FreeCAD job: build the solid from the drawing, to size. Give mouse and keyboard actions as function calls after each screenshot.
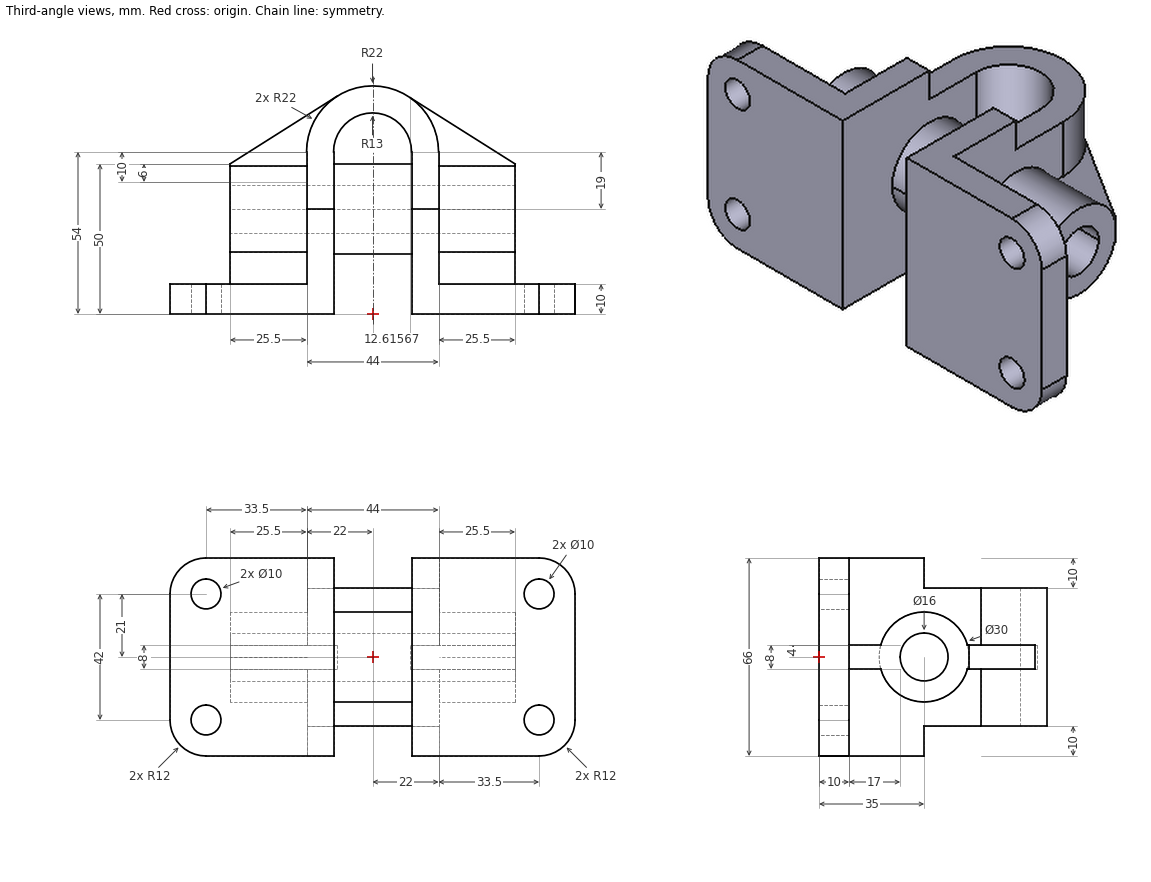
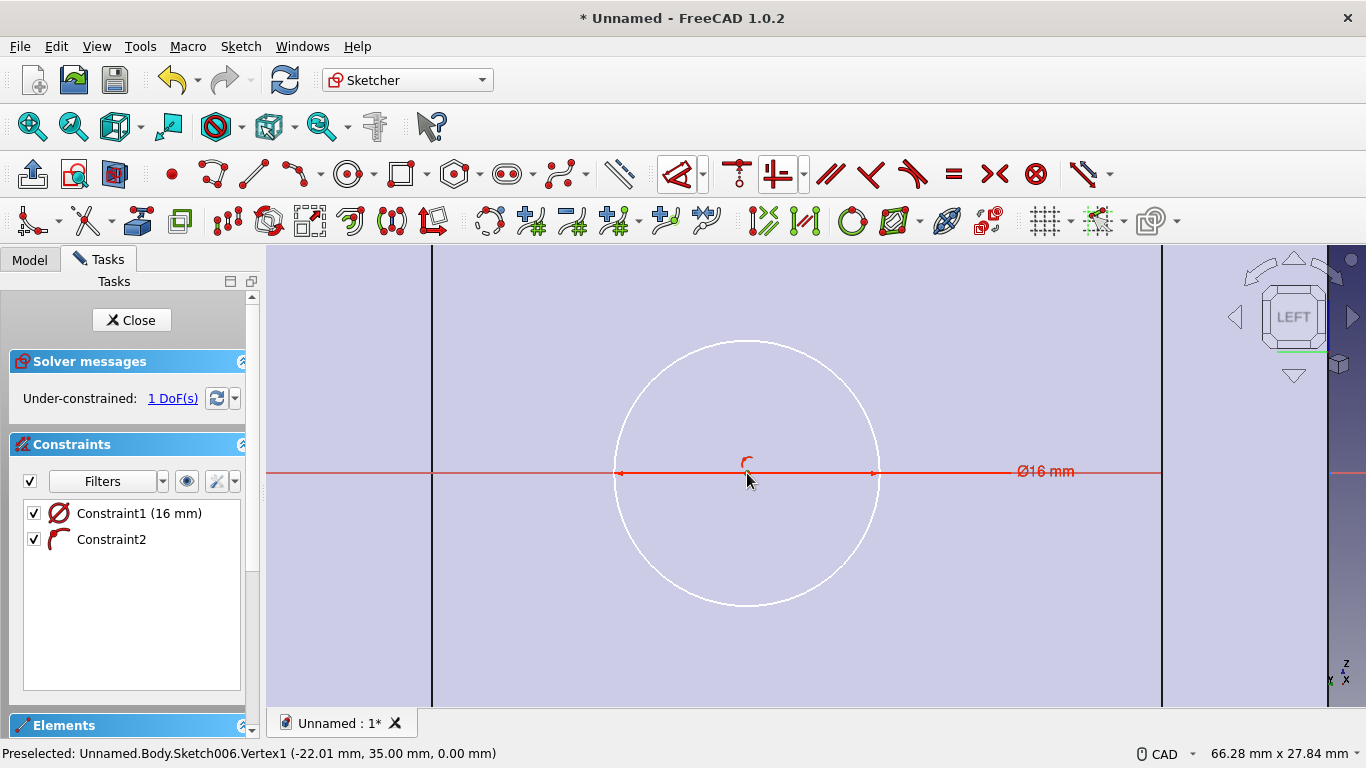
click(702, 174)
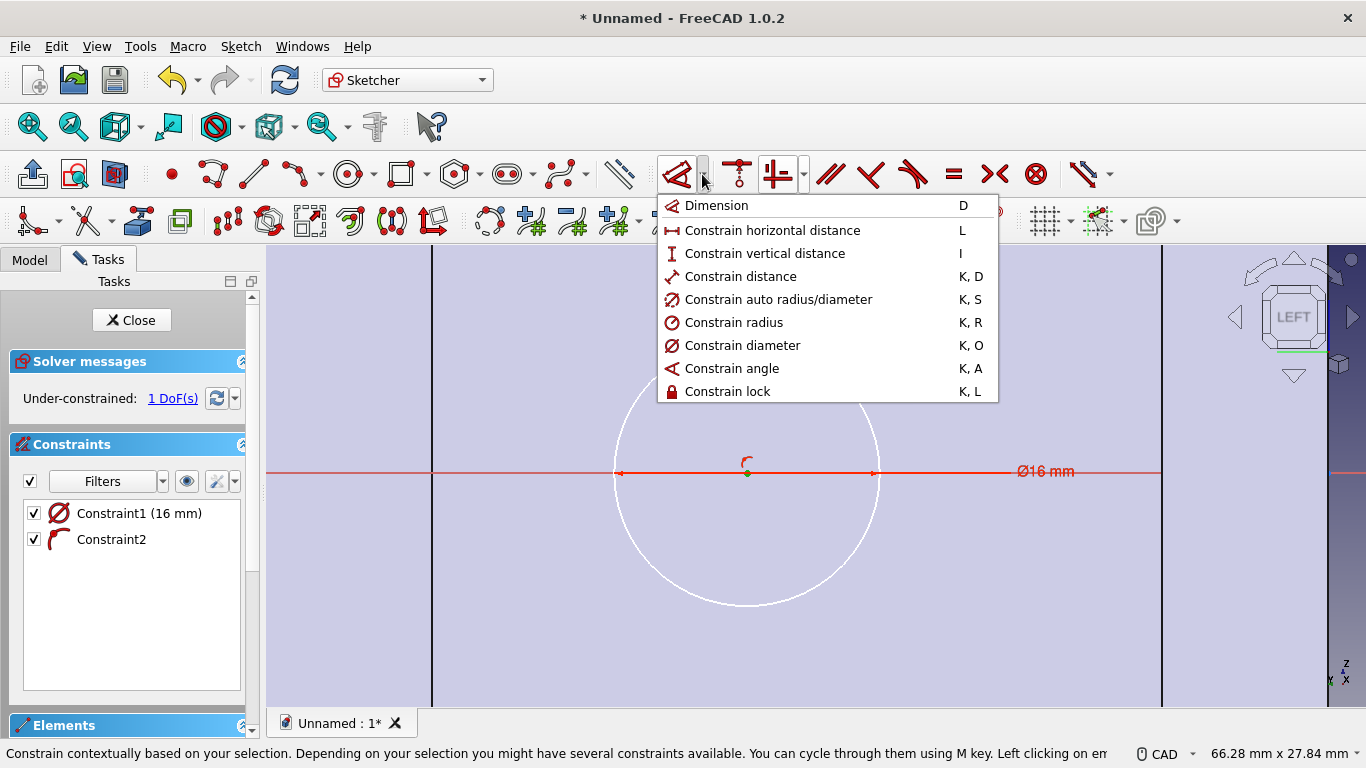
click(828, 230)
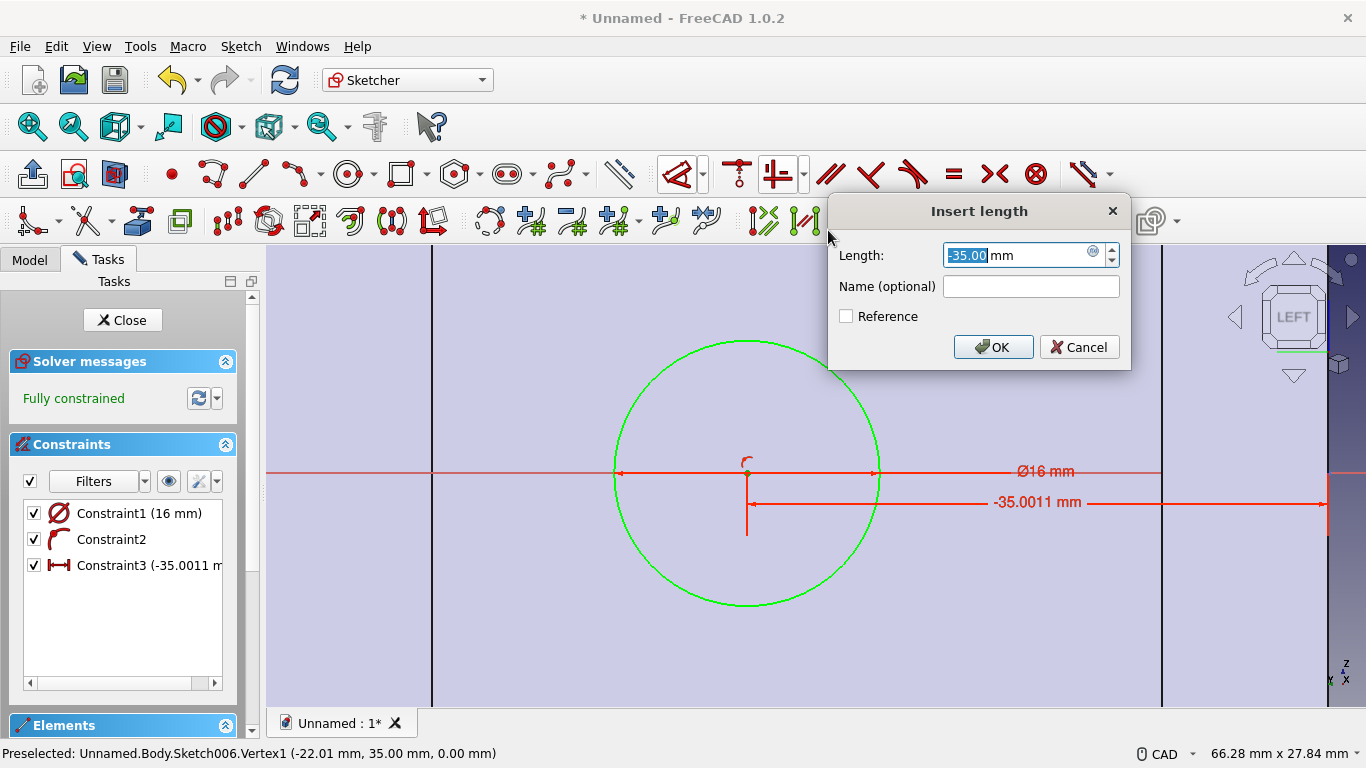
text(-35)
key(Return)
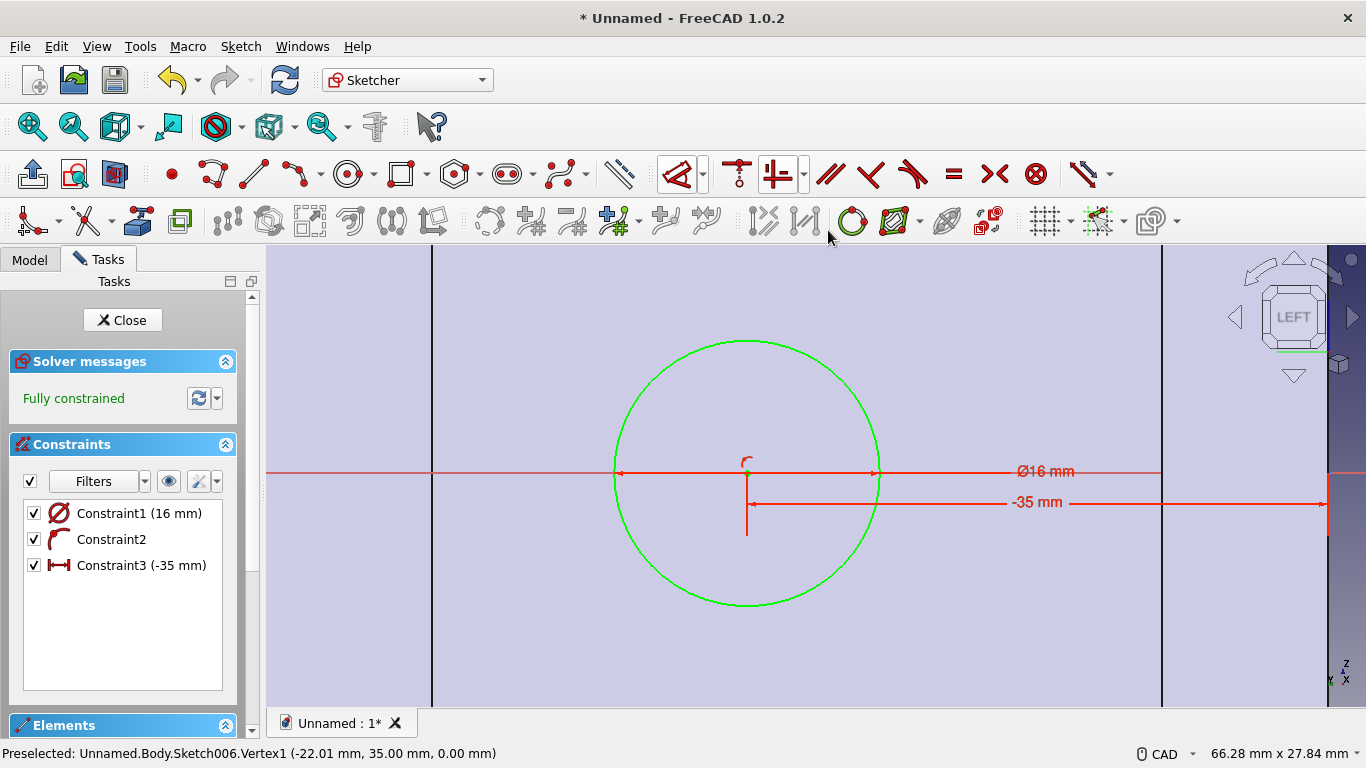
click(123, 320)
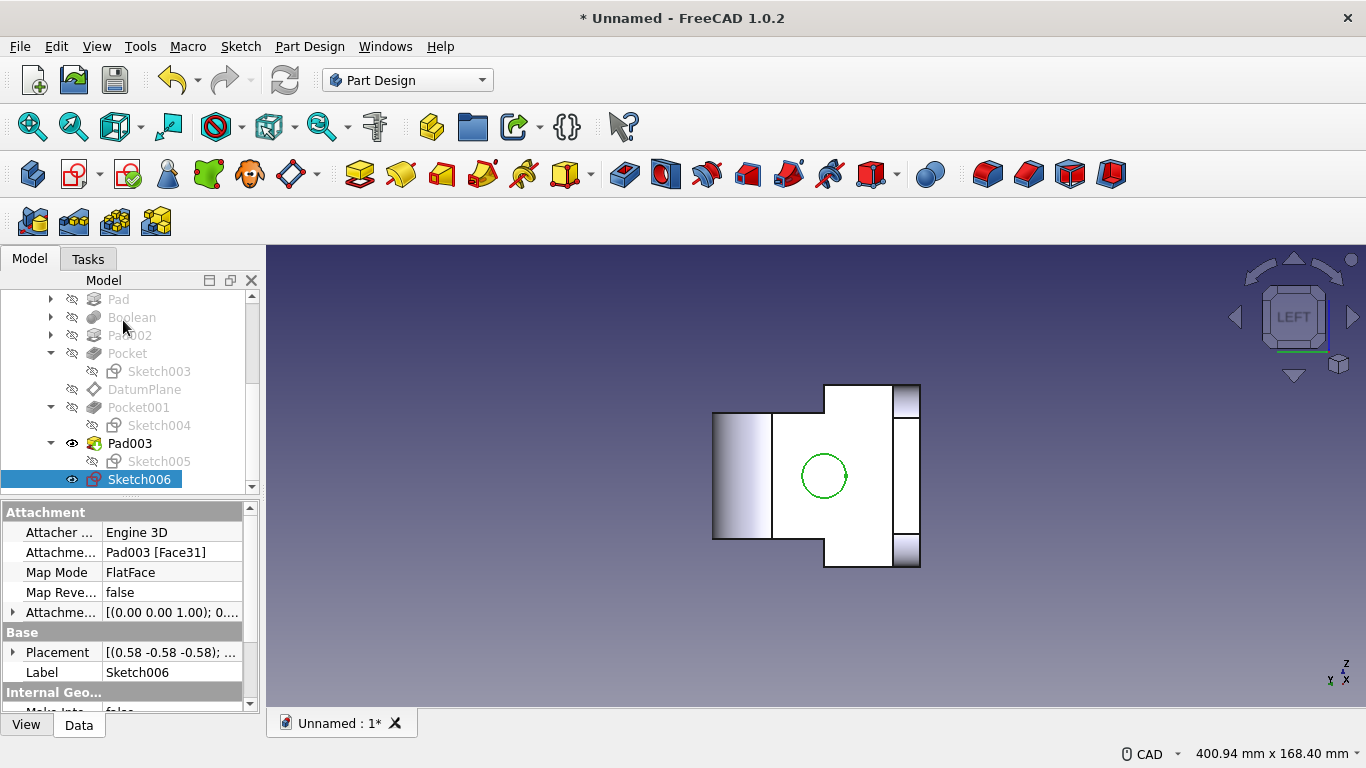
click(625, 174)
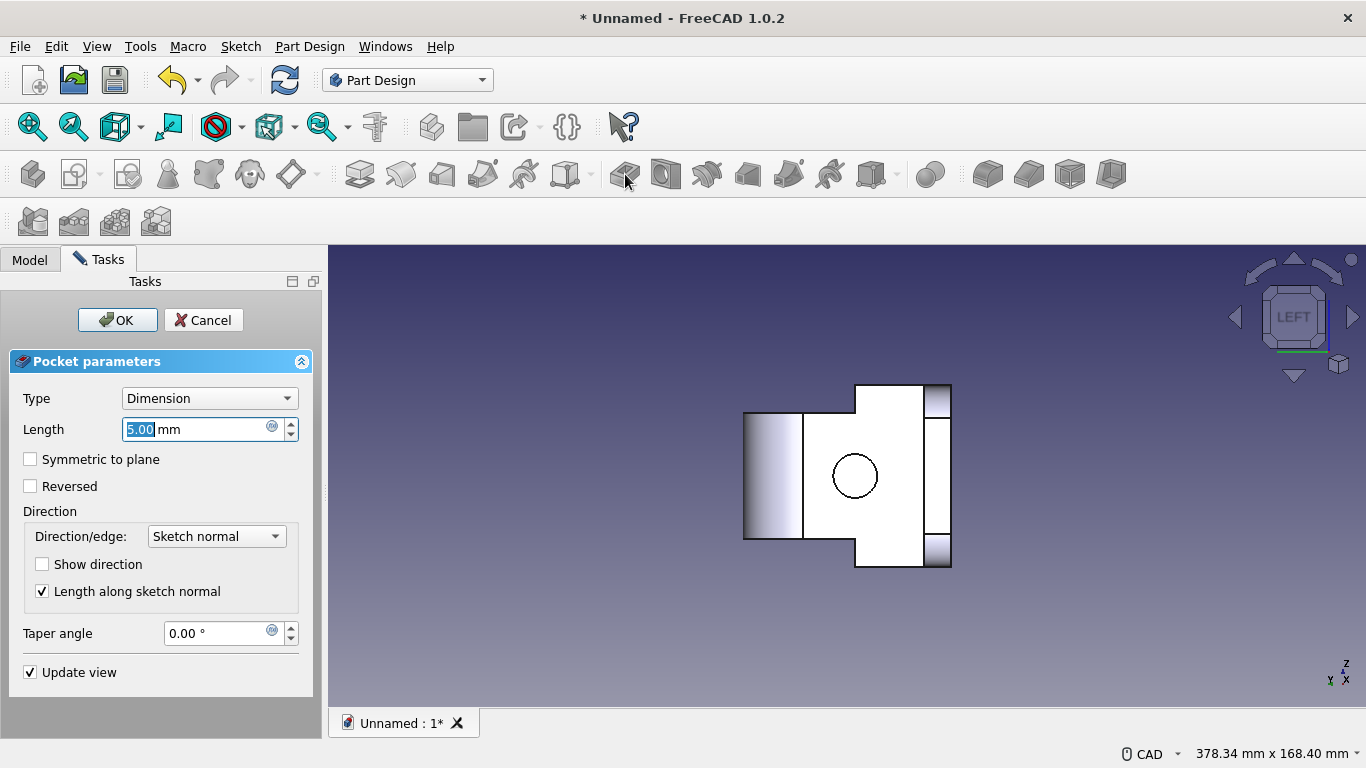
text(44)
key(Tab)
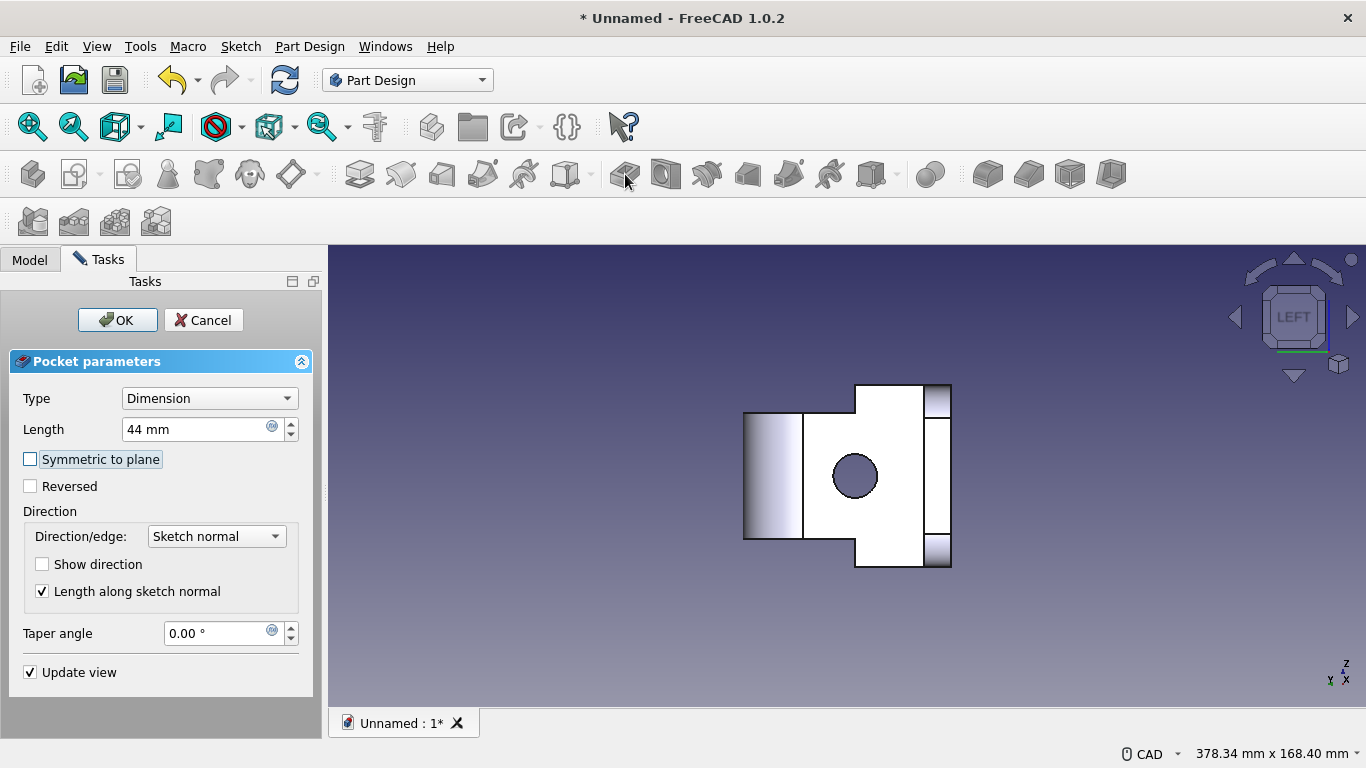
click(118, 320)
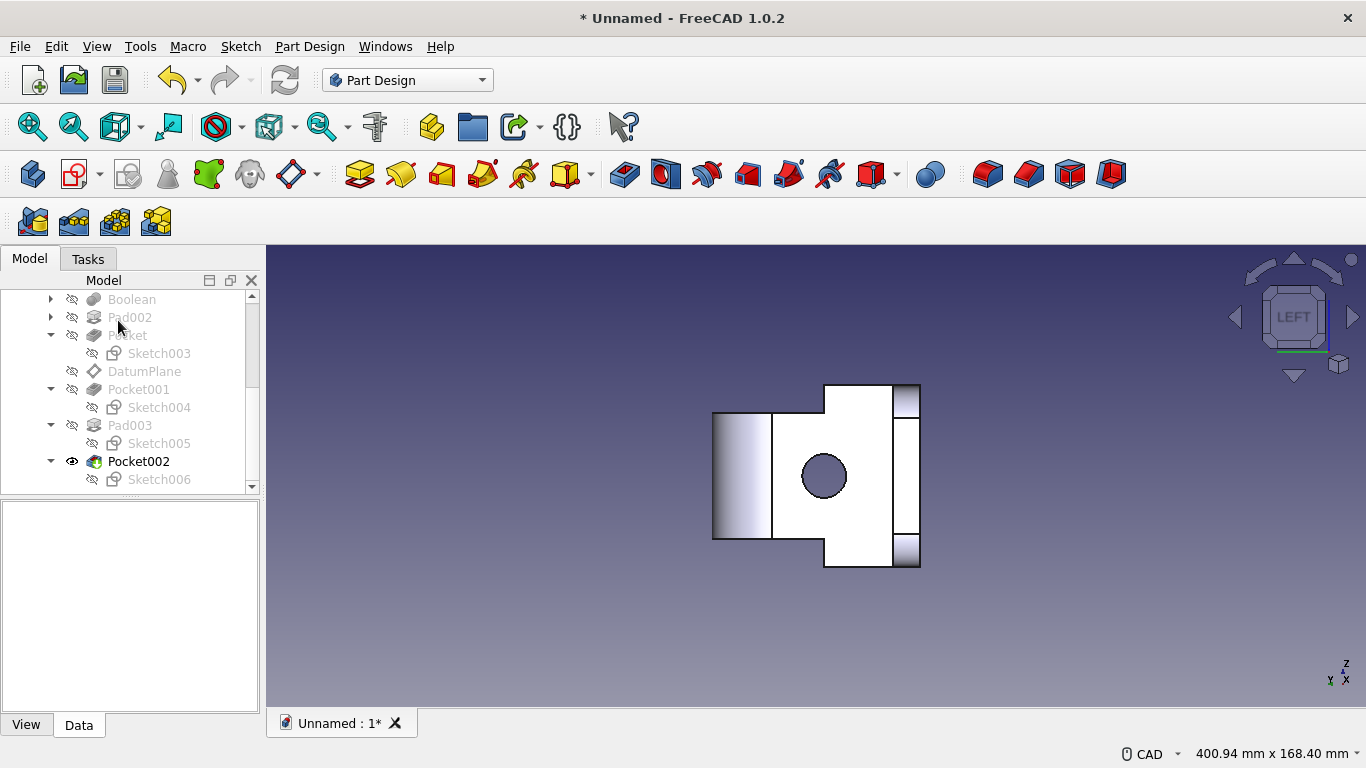
click(33, 128)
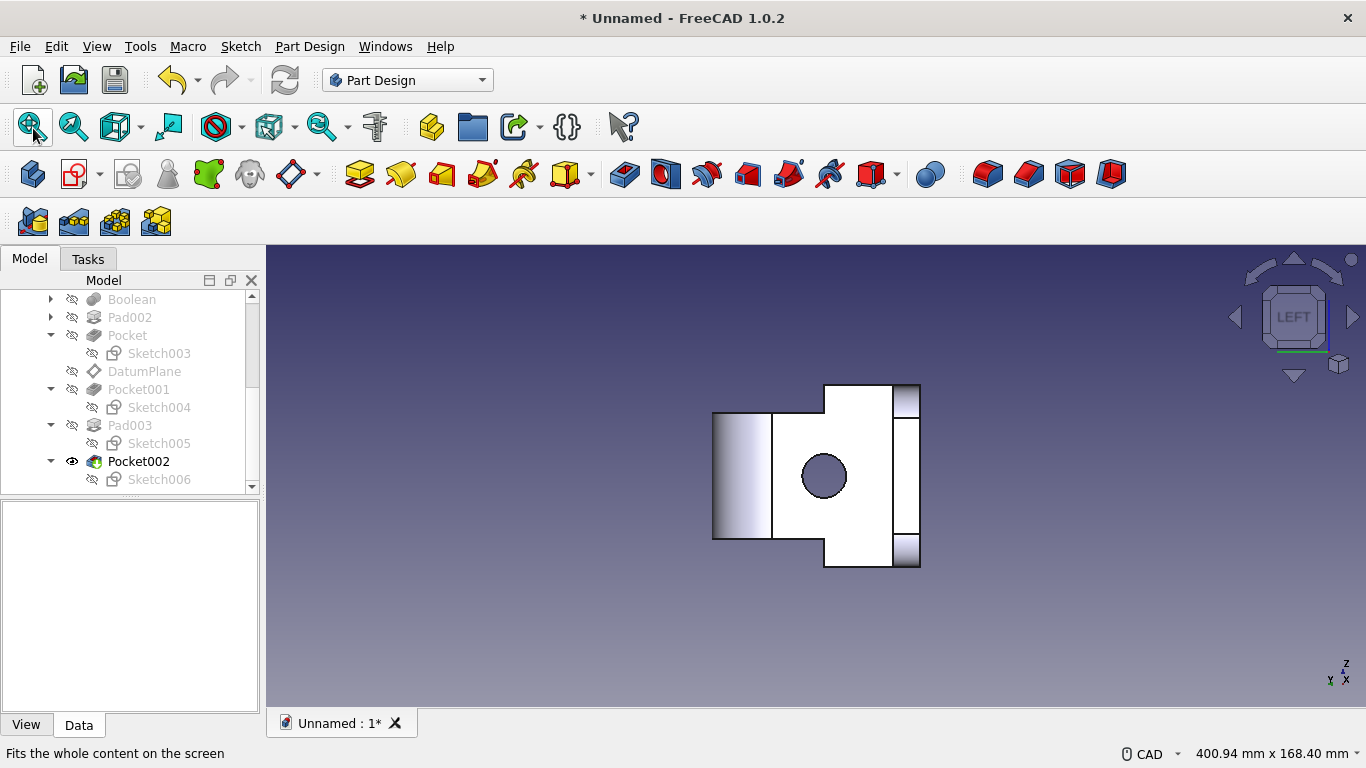
scroll(141, 385, down, 3)